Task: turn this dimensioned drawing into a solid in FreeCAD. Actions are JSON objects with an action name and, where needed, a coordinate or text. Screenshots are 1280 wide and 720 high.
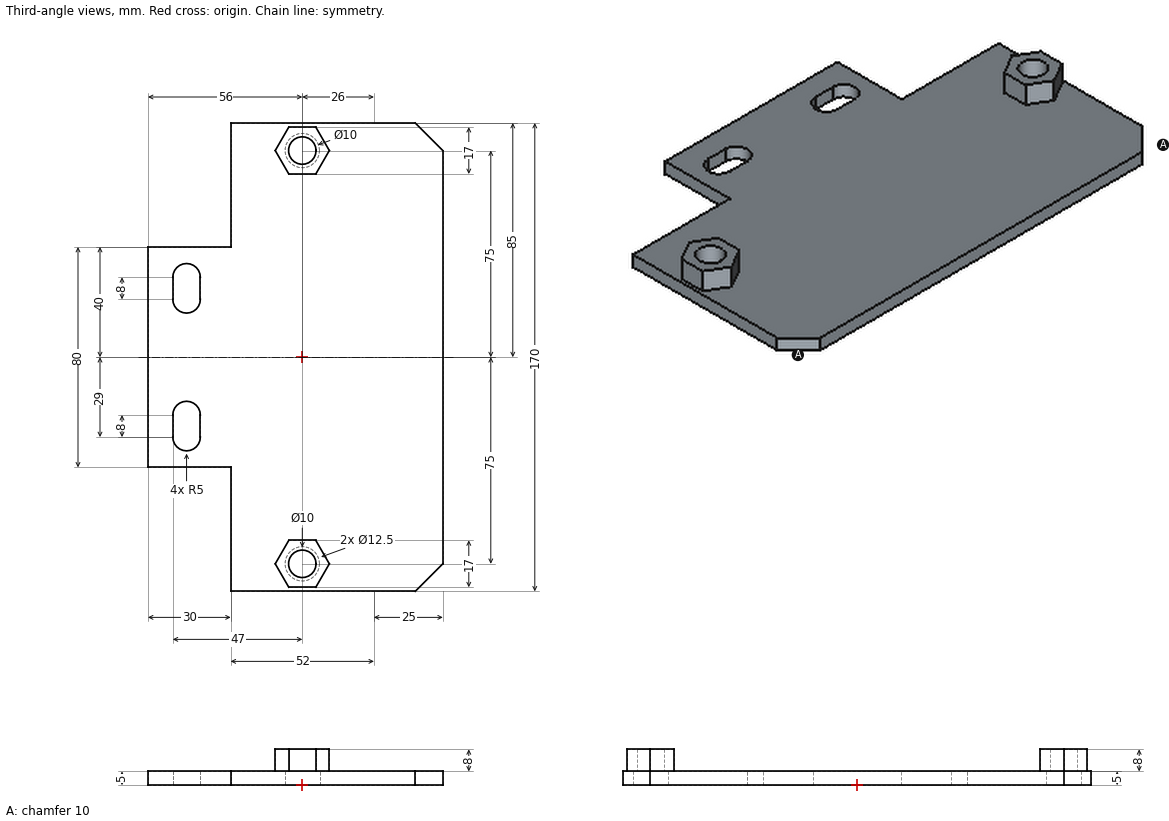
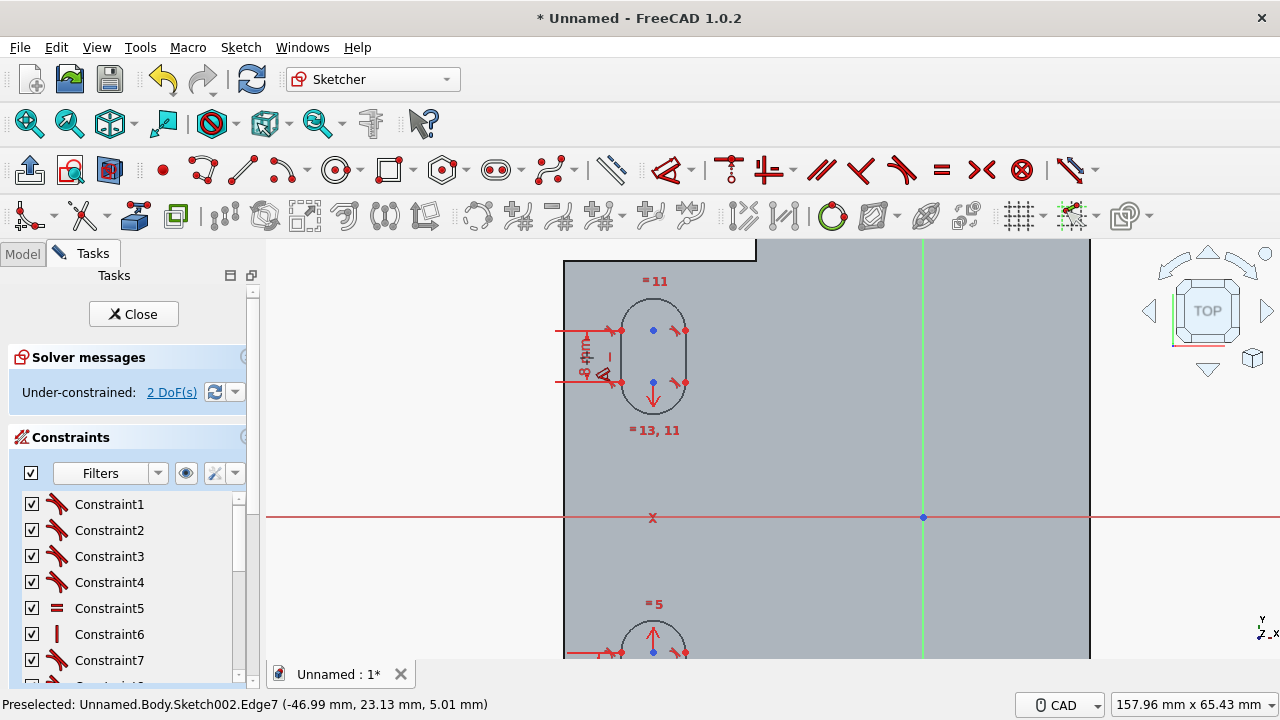
{"action": "scroll", "coordinate": [622, 366], "scroll_direction": "down", "scroll_amount": 3}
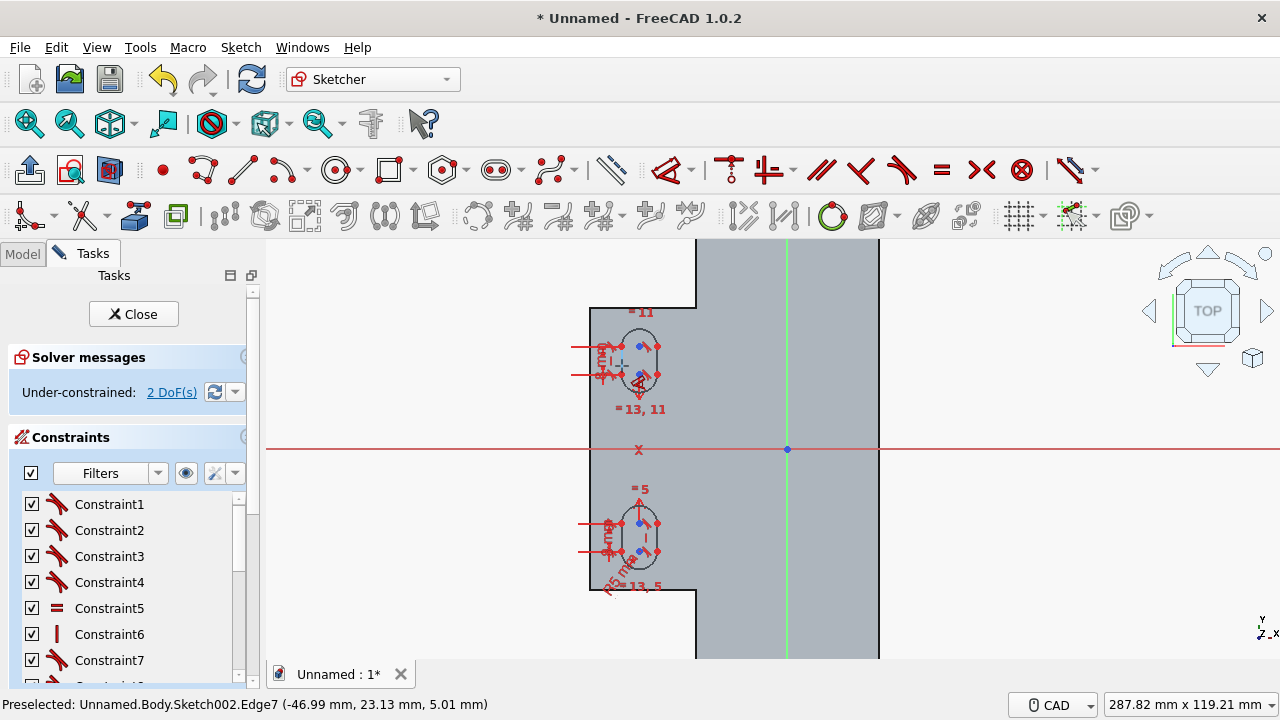
{"action": "left_click", "coordinate": [622, 552]}
{"action": "left_click", "coordinate": [705, 586]}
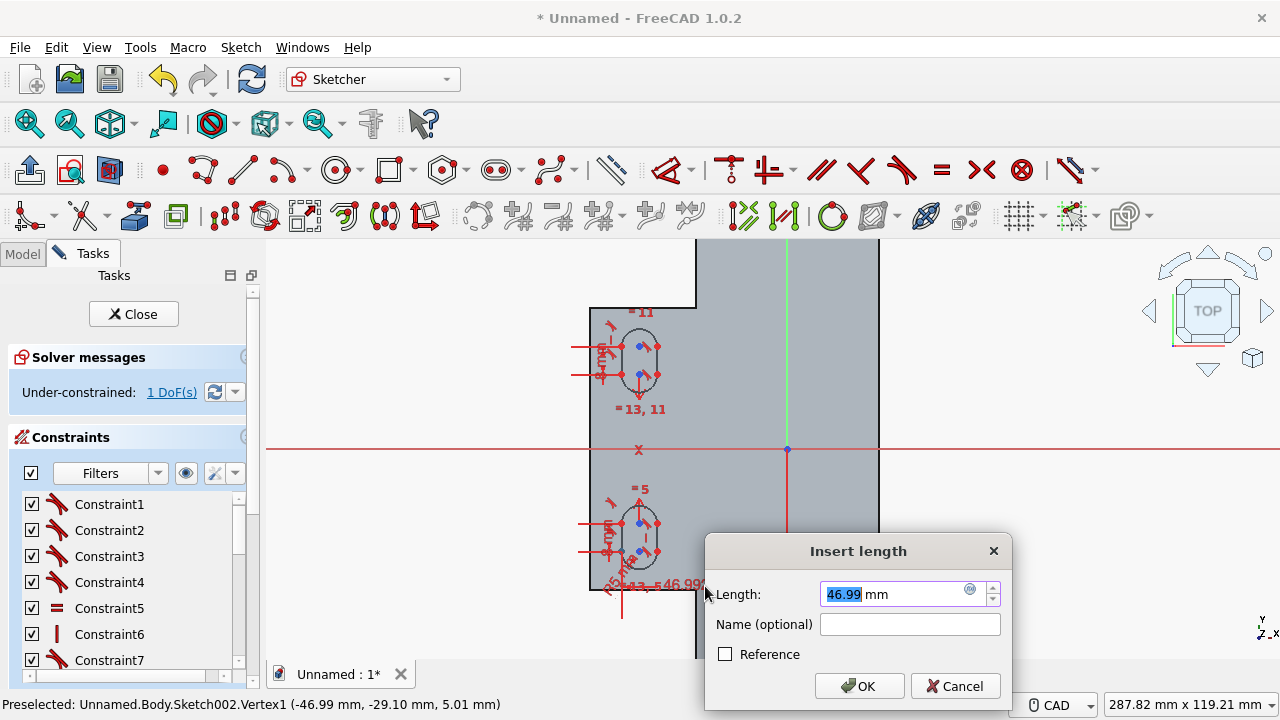
{"action": "type", "text": "47"}
{"action": "key", "text": "Return"}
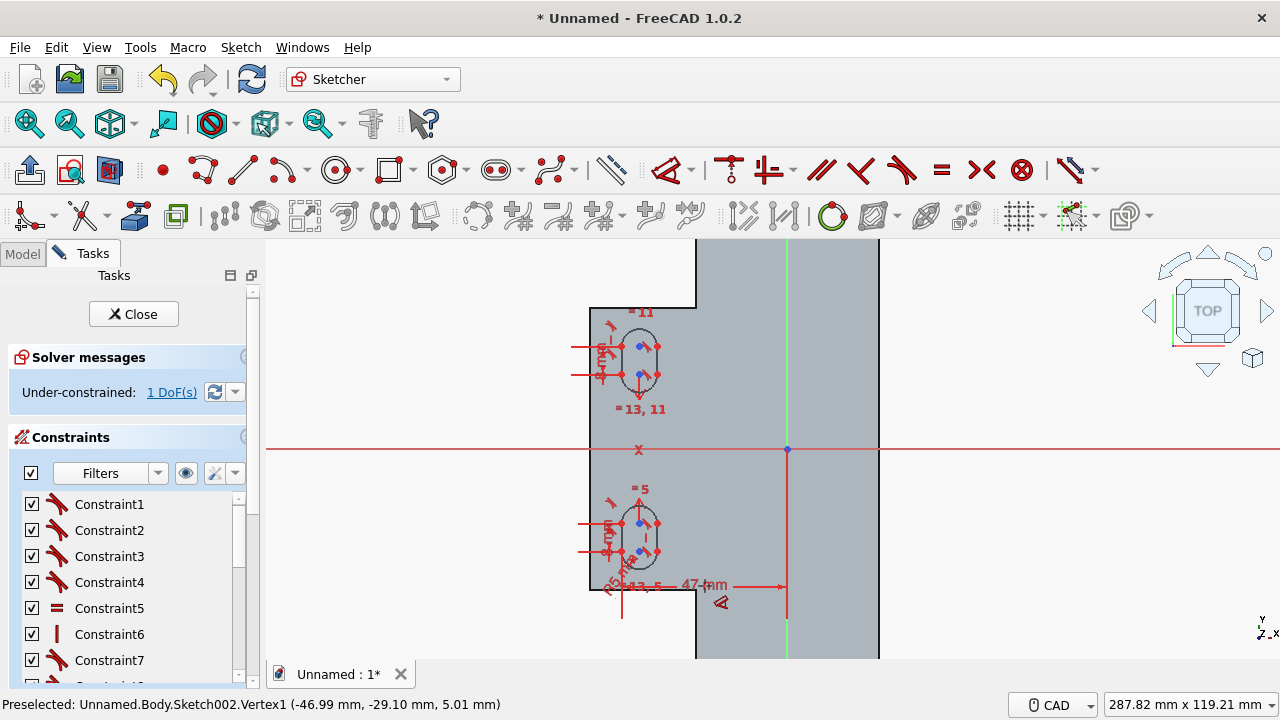
{"action": "left_click", "coordinate": [622, 552]}
{"action": "left_click", "coordinate": [821, 501]}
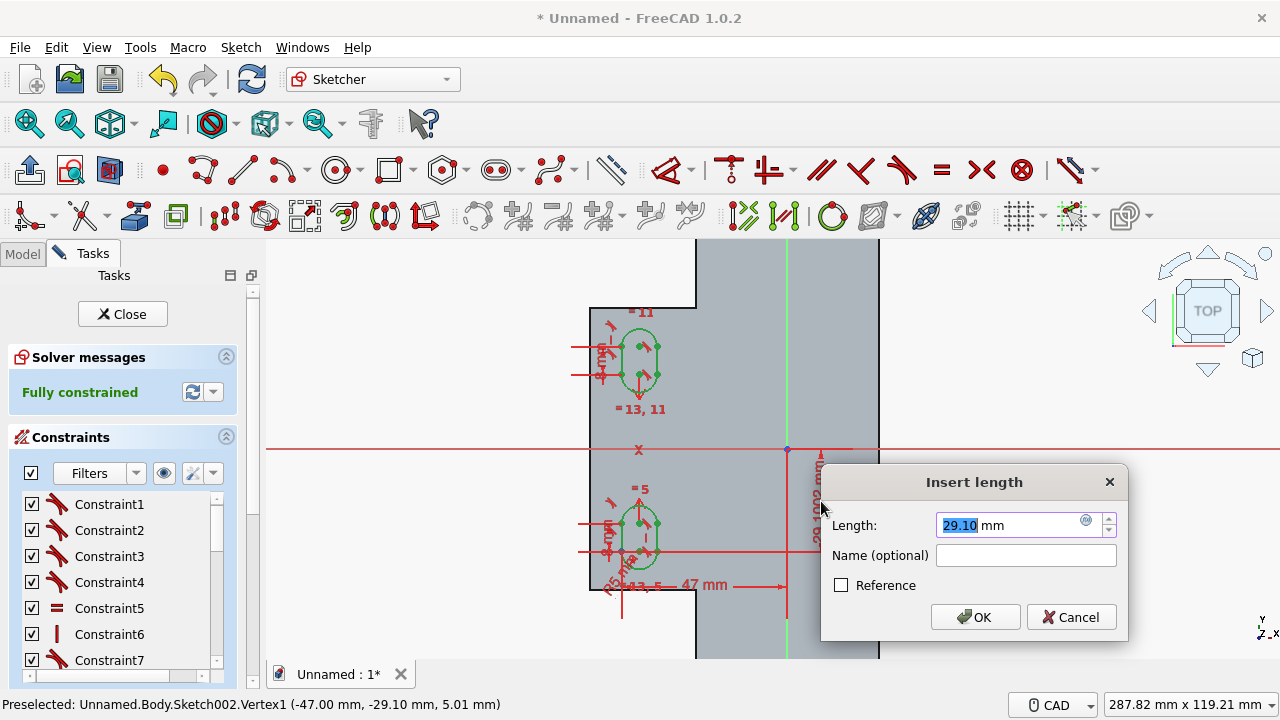
{"action": "type", "text": "29"}
{"action": "key", "text": "Return"}
{"action": "key", "text": "Escape"}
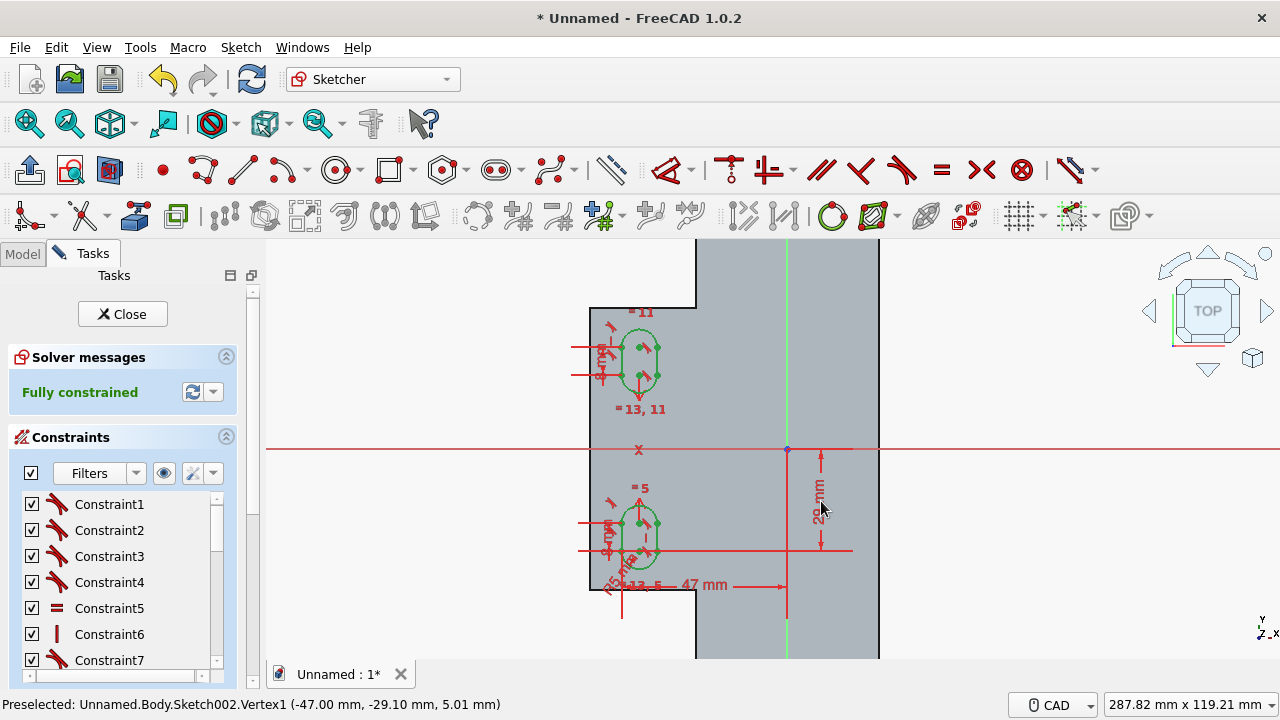
{"action": "left_click", "coordinate": [123, 314]}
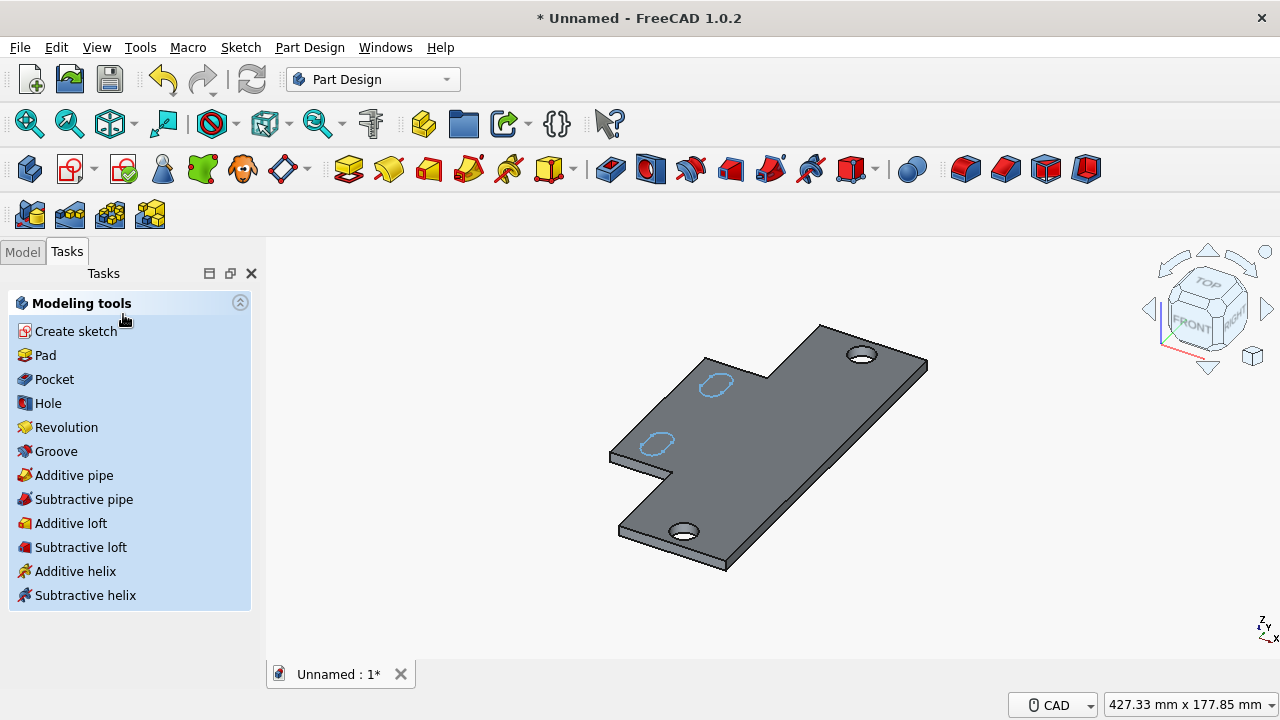
{"action": "left_click", "coordinate": [612, 170]}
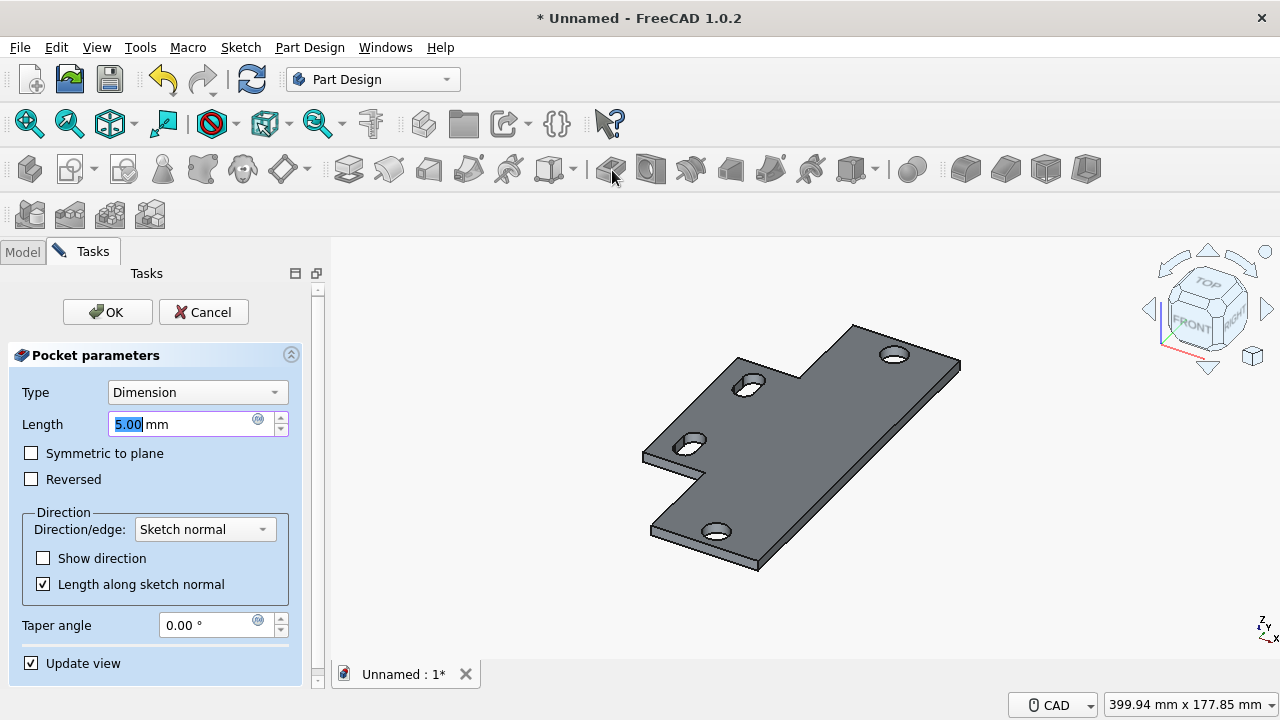
{"action": "left_click", "coordinate": [198, 392]}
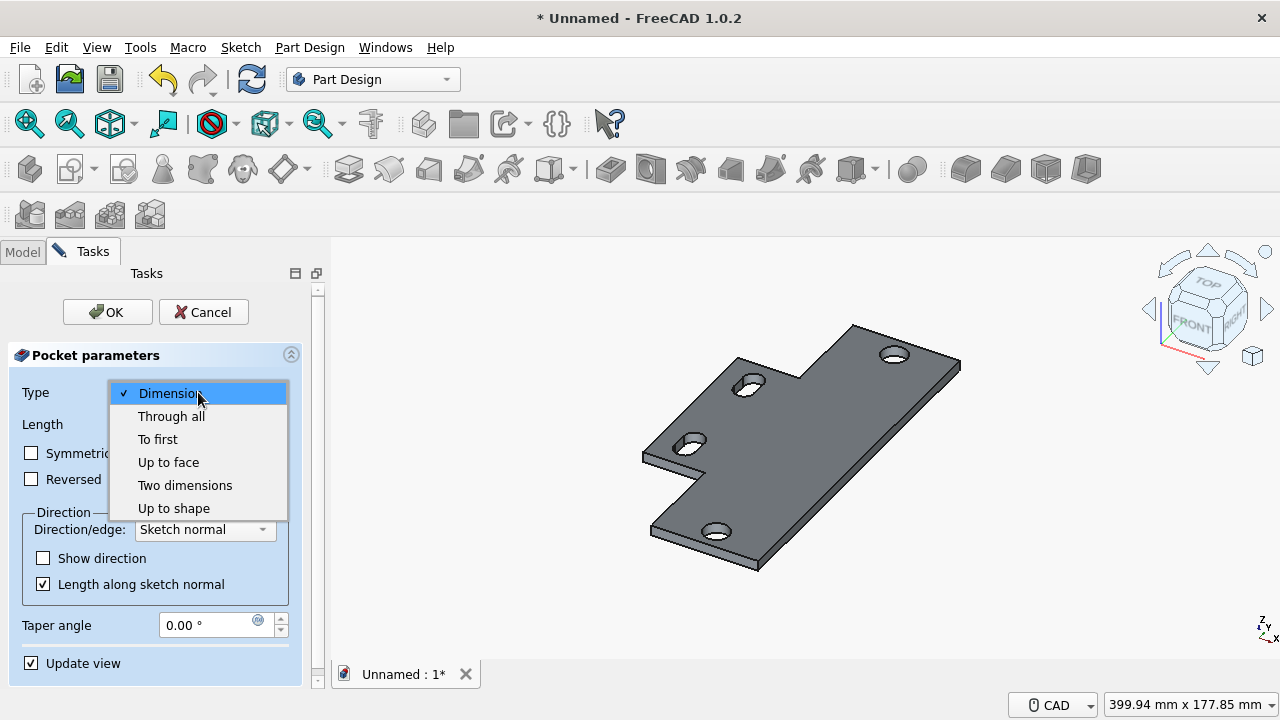
{"action": "left_click", "coordinate": [198, 416]}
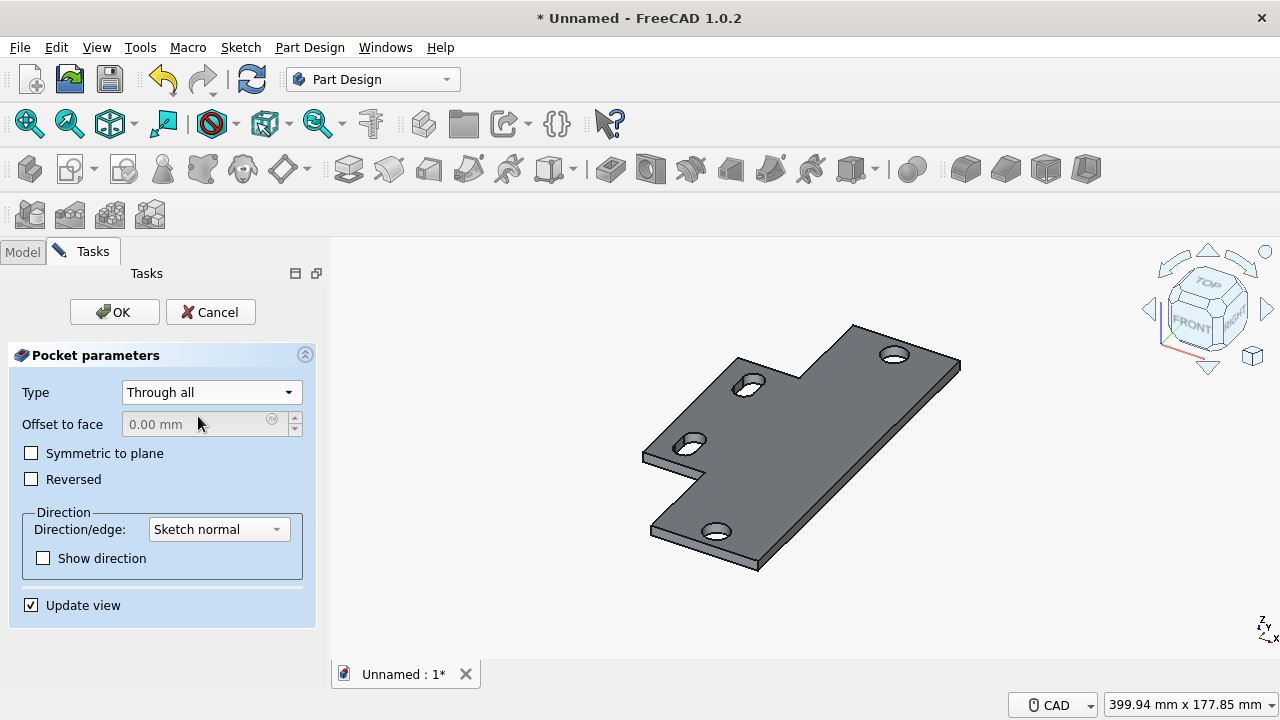
{"action": "left_click", "coordinate": [115, 312]}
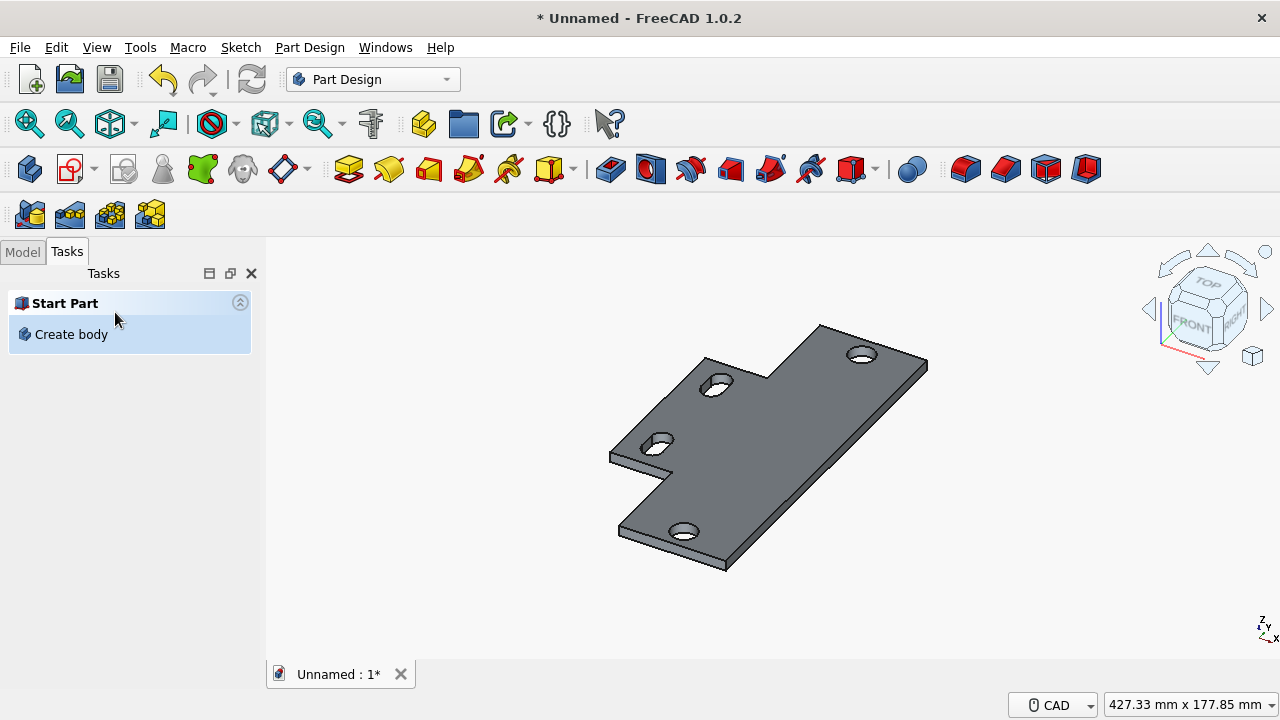
{"action": "left_click", "coordinate": [30, 170]}